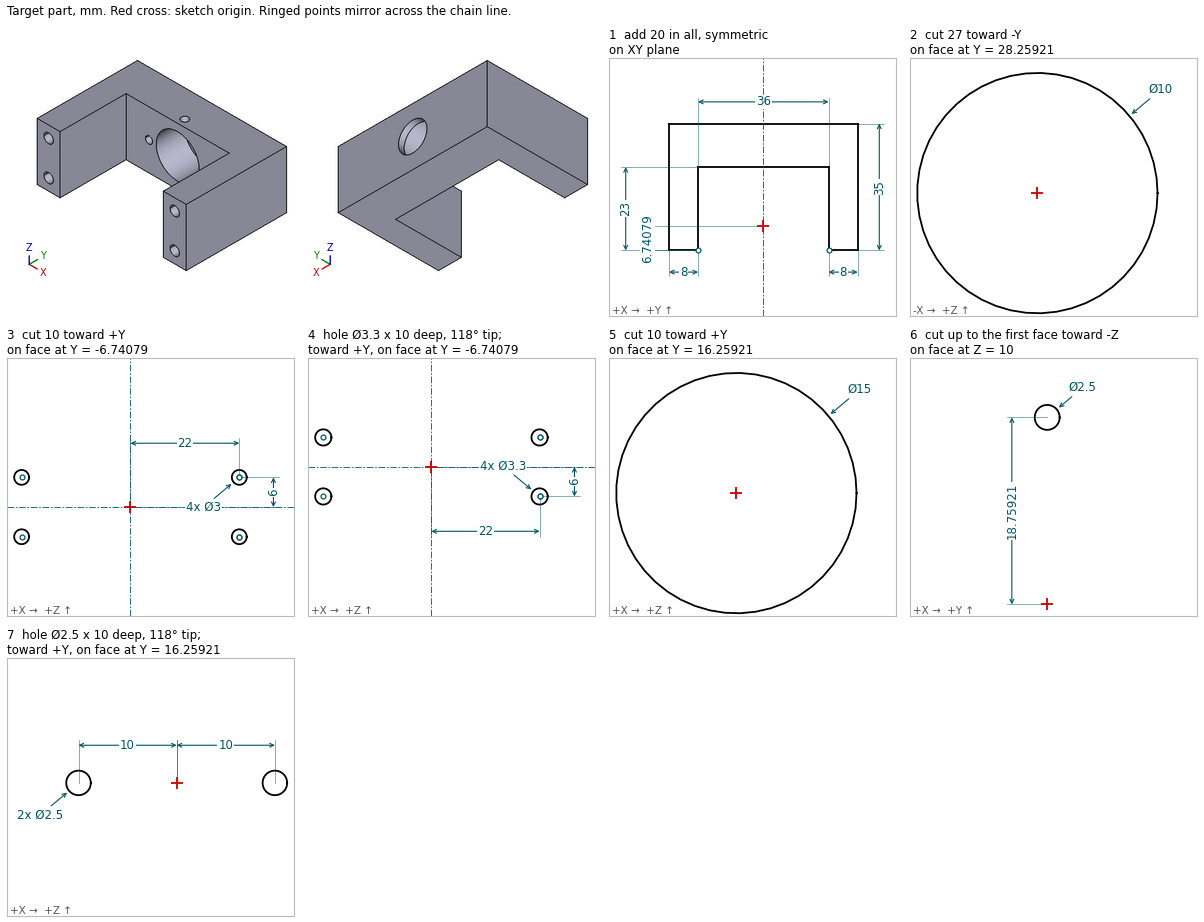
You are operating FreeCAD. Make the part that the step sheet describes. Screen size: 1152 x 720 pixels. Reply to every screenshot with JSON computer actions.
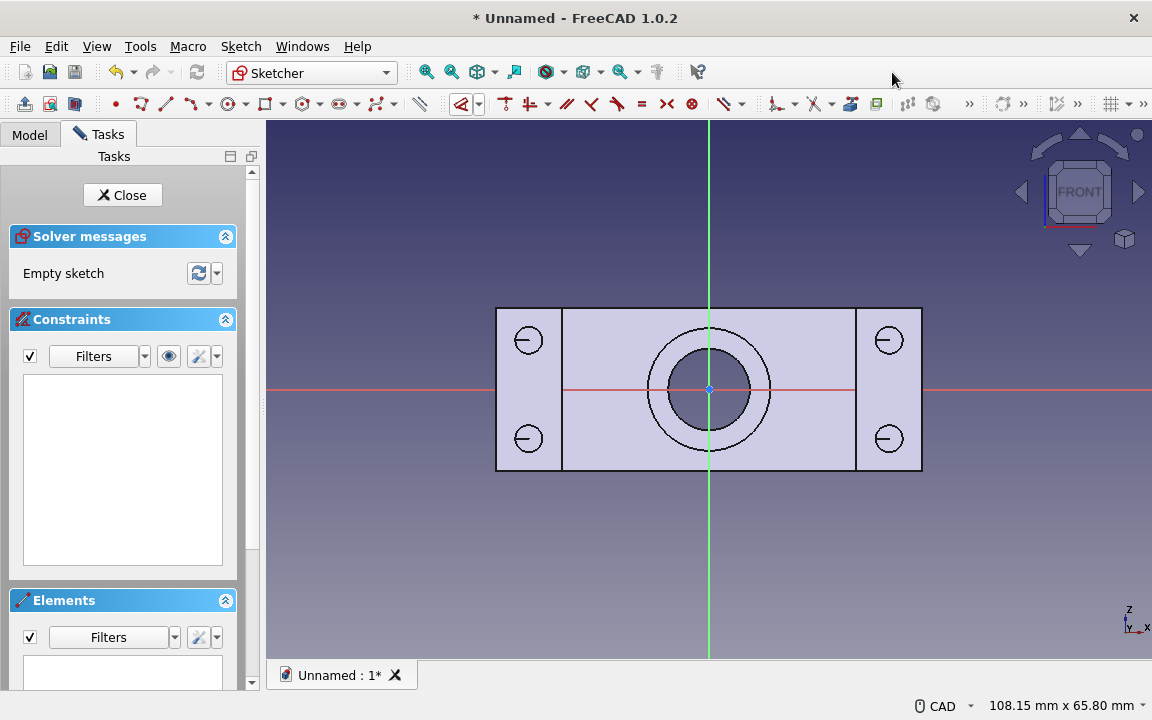
{"action": "key", "text": "q s"}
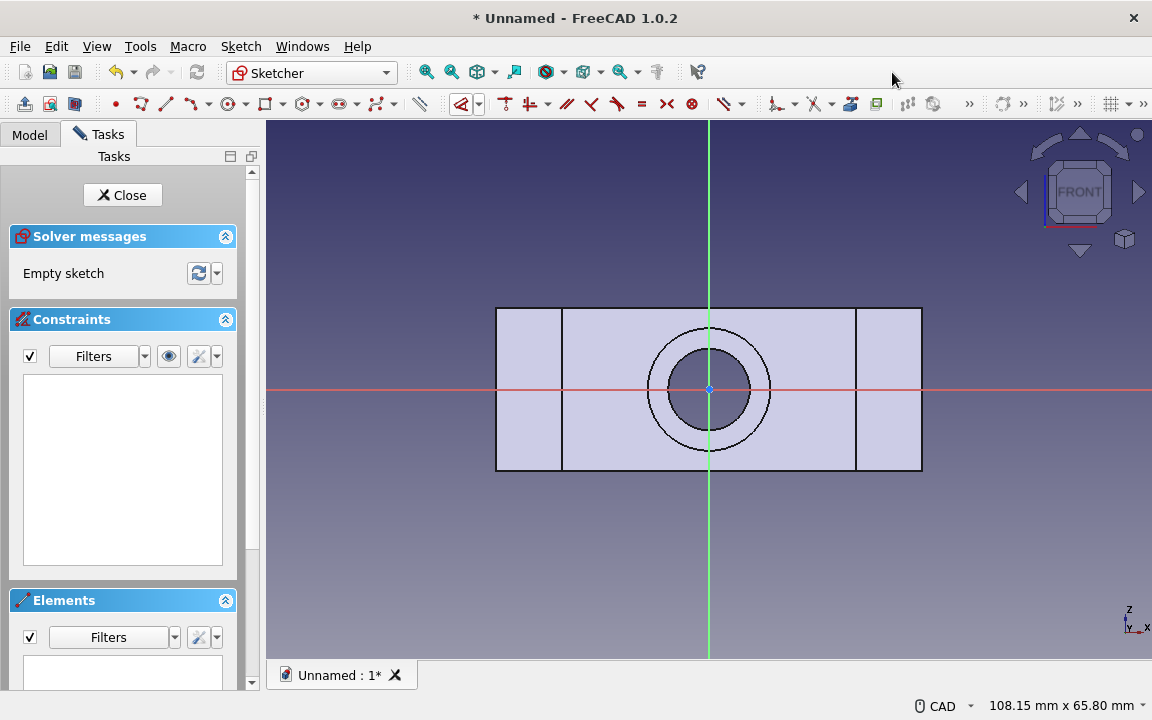
{"action": "scroll", "coordinate": [749, 390], "scroll_direction": "up", "scroll_amount": 5}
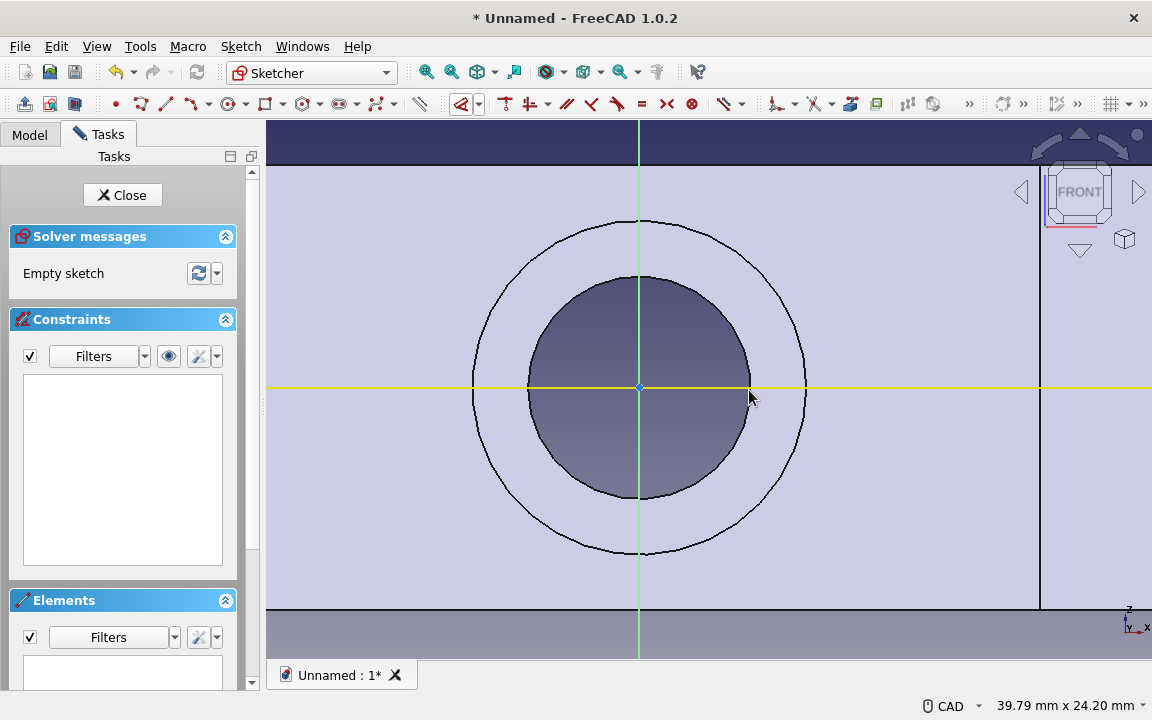
{"action": "key", "text": "g c"}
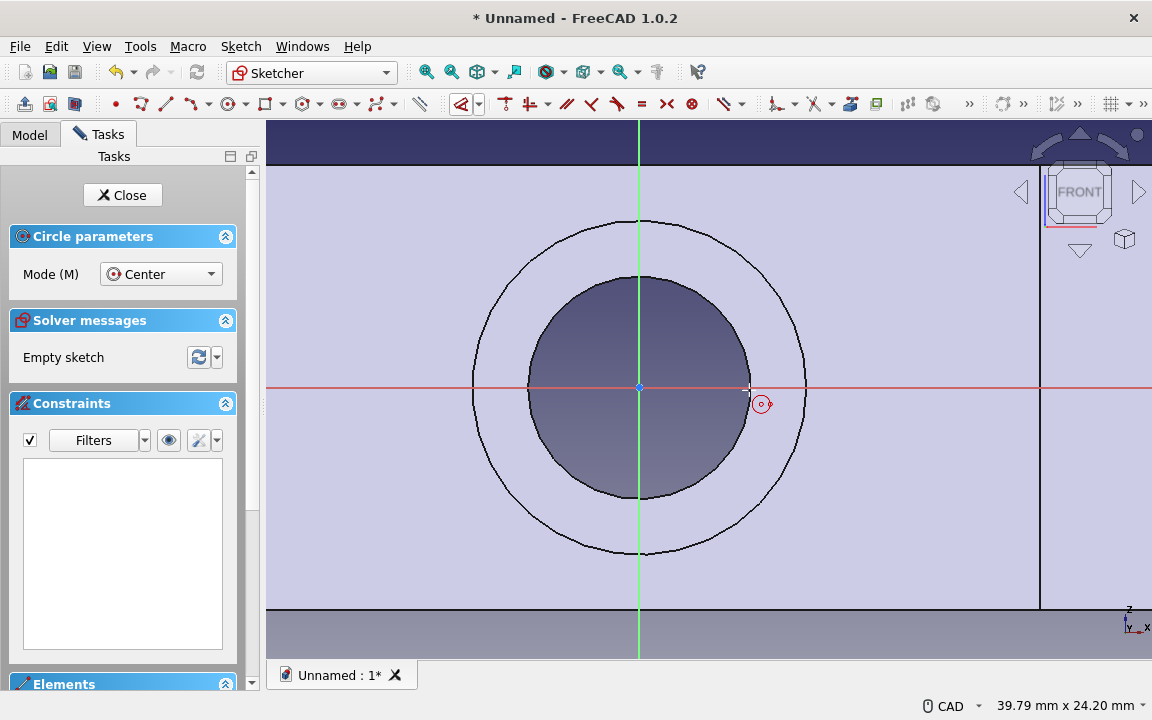
{"action": "left_click", "coordinate": [417, 388]}
{"action": "left_click", "coordinate": [436, 368]}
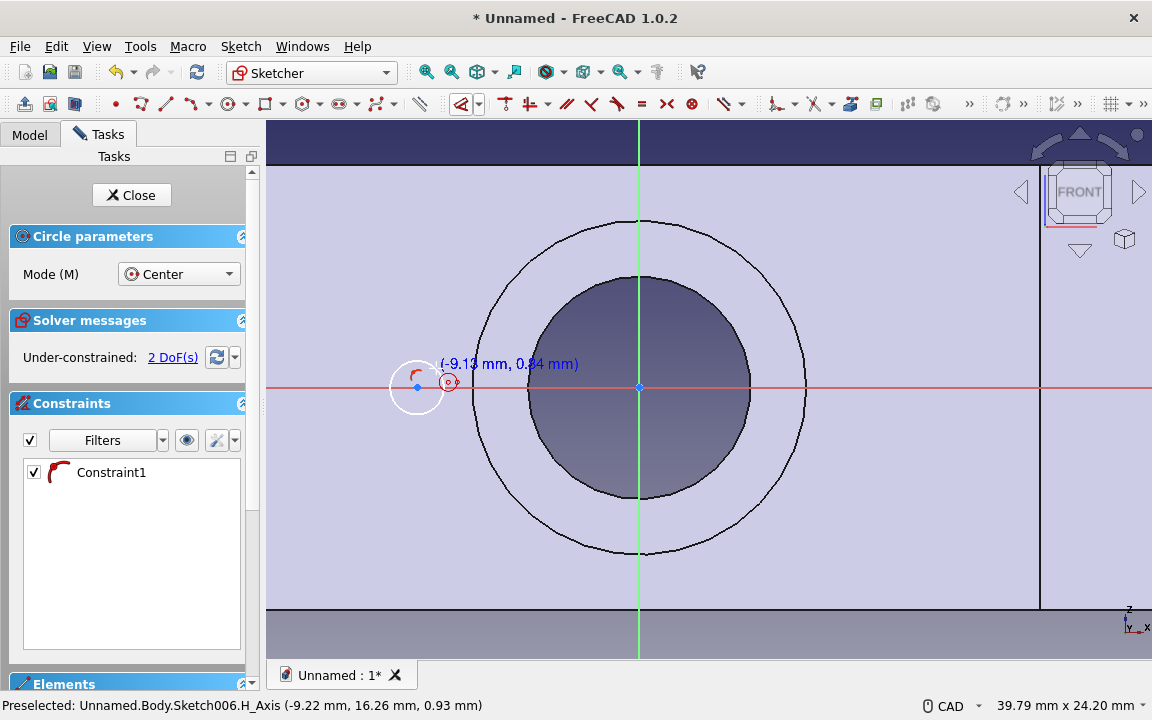
{"action": "left_click", "coordinate": [862, 388]}
{"action": "left_click", "coordinate": [882, 368]}
{"action": "key", "text": "Escape"}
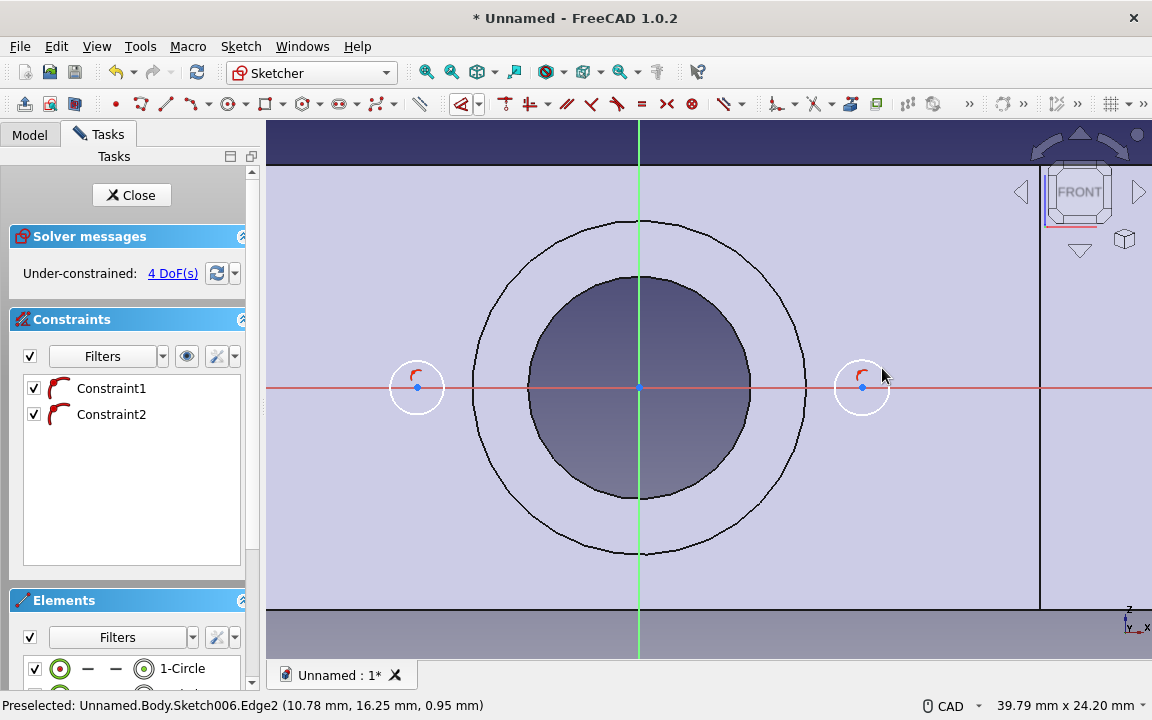
{"action": "left_click", "coordinate": [436, 369]}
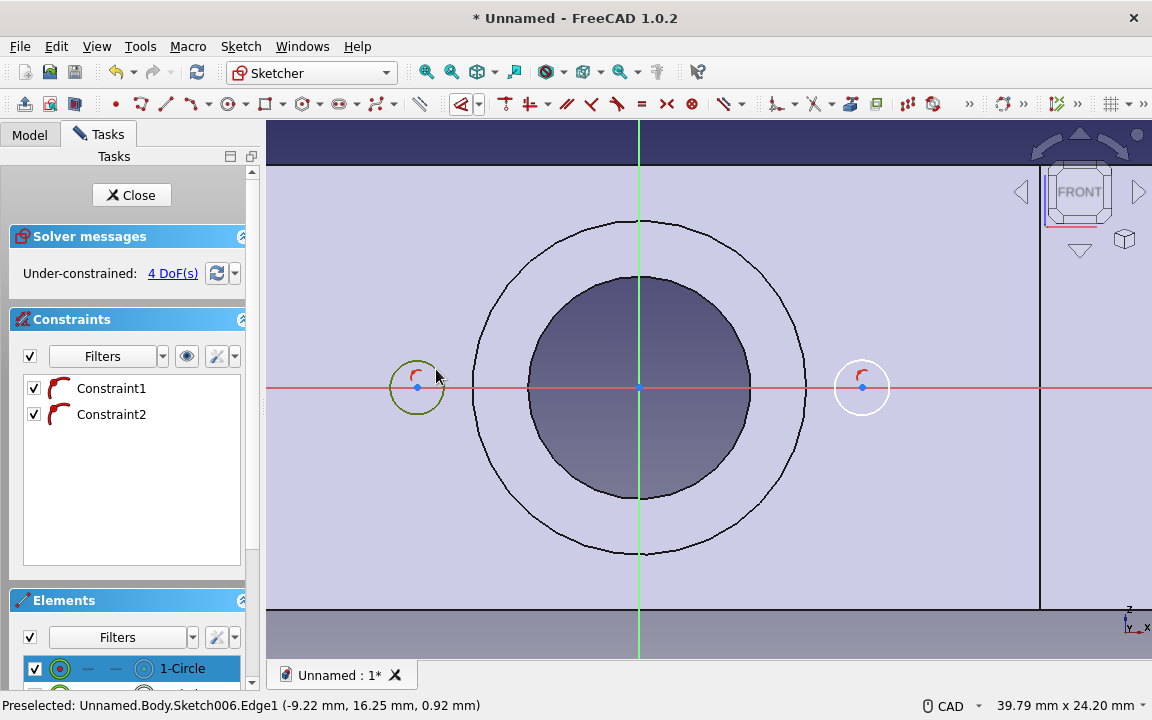
{"action": "left_click", "coordinate": [881, 368]}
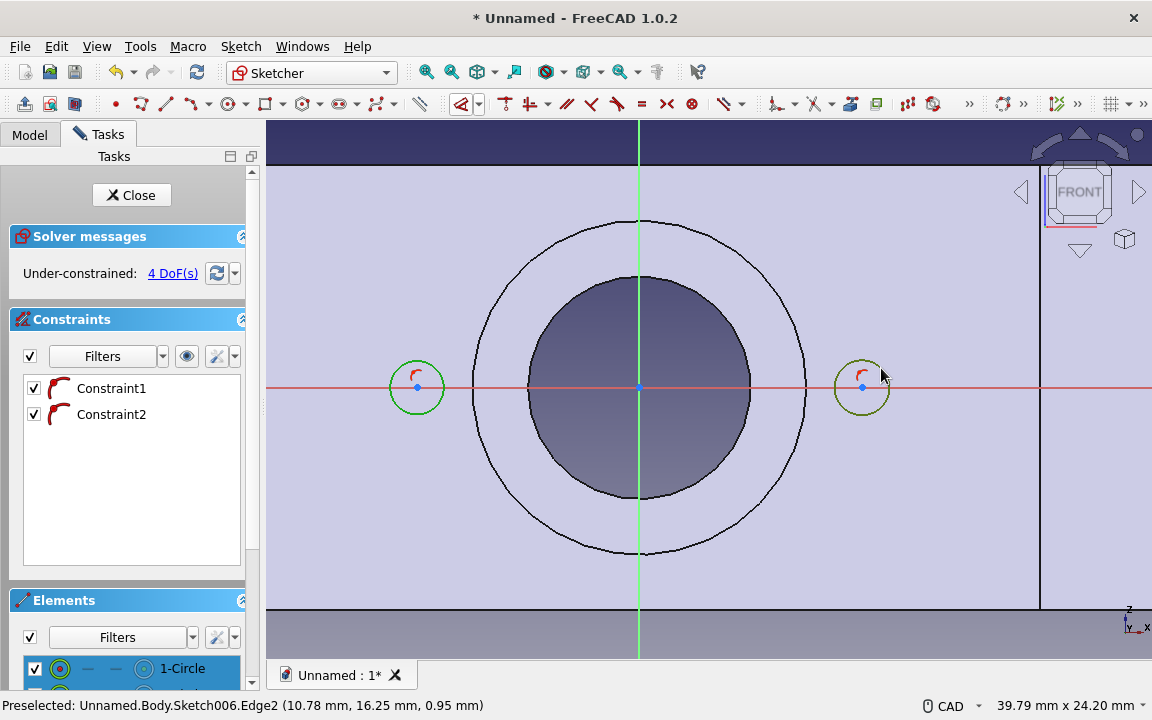
{"action": "key", "text": "e"}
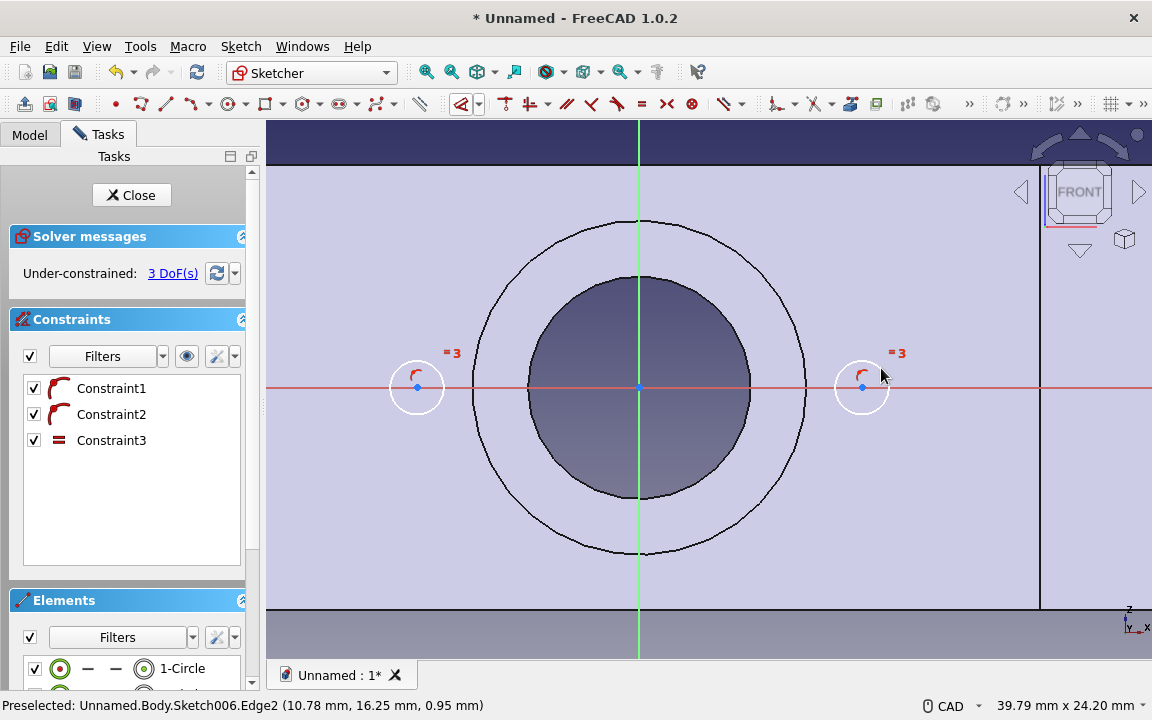
{"action": "left_click", "coordinate": [436, 369]}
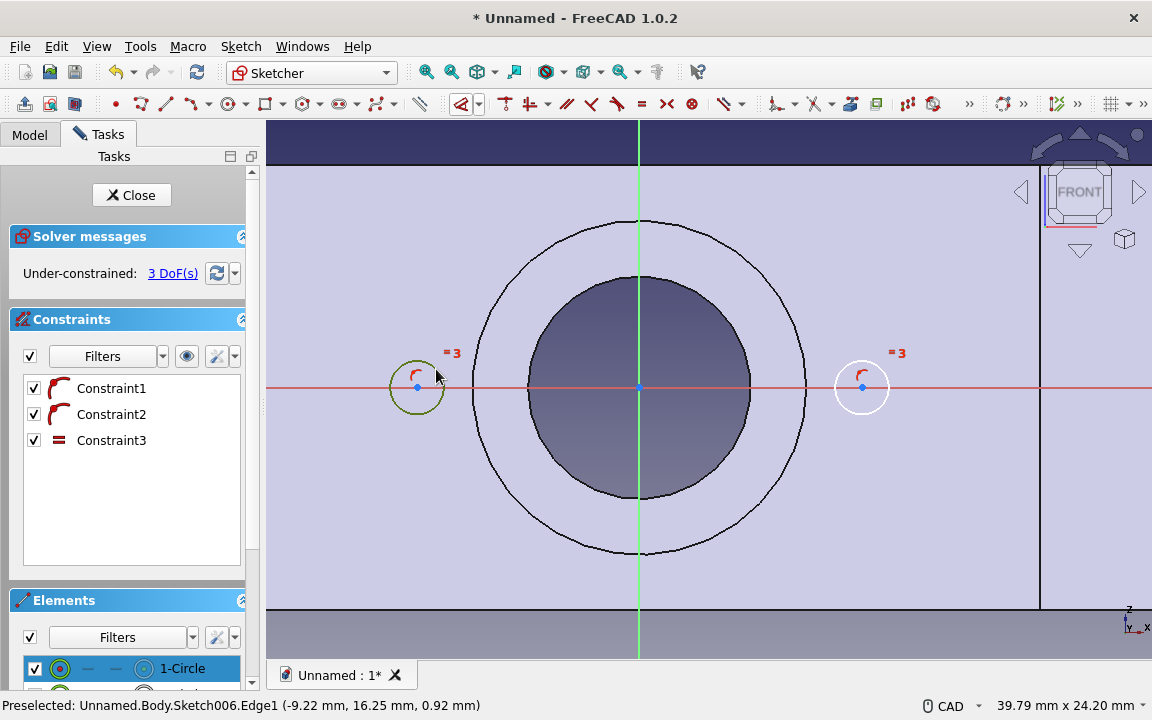
{"action": "key", "text": "k o"}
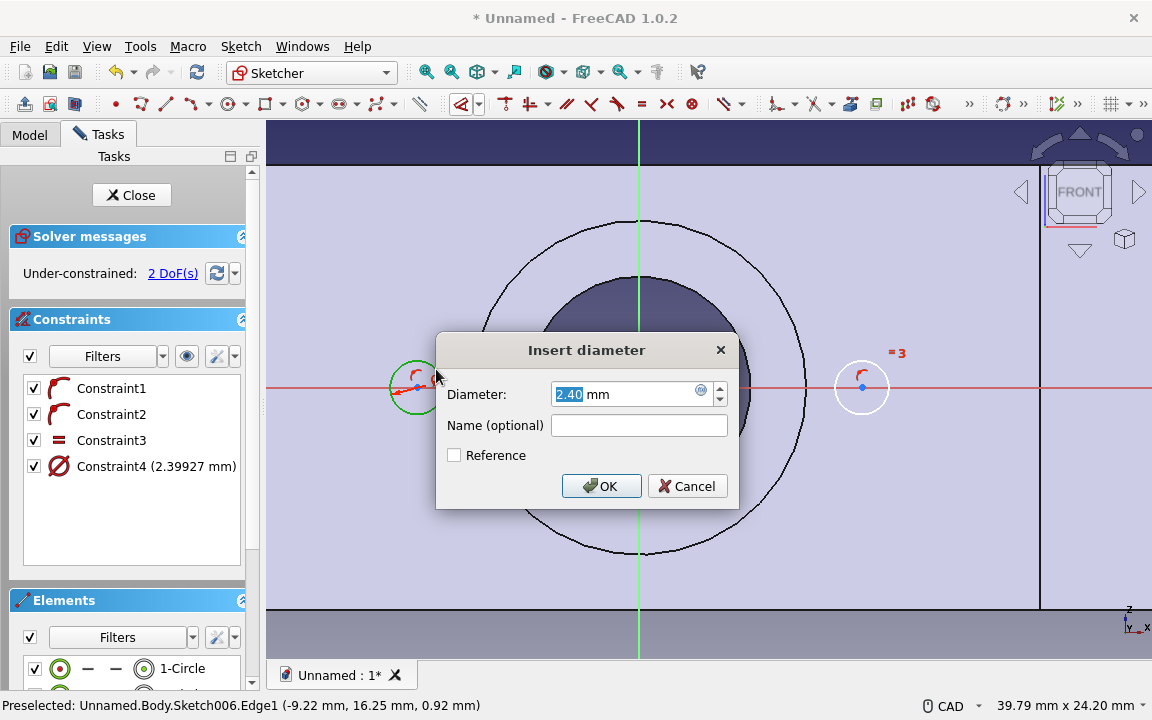
{"action": "type", "text": "2.5"}
{"action": "key", "text": "Return"}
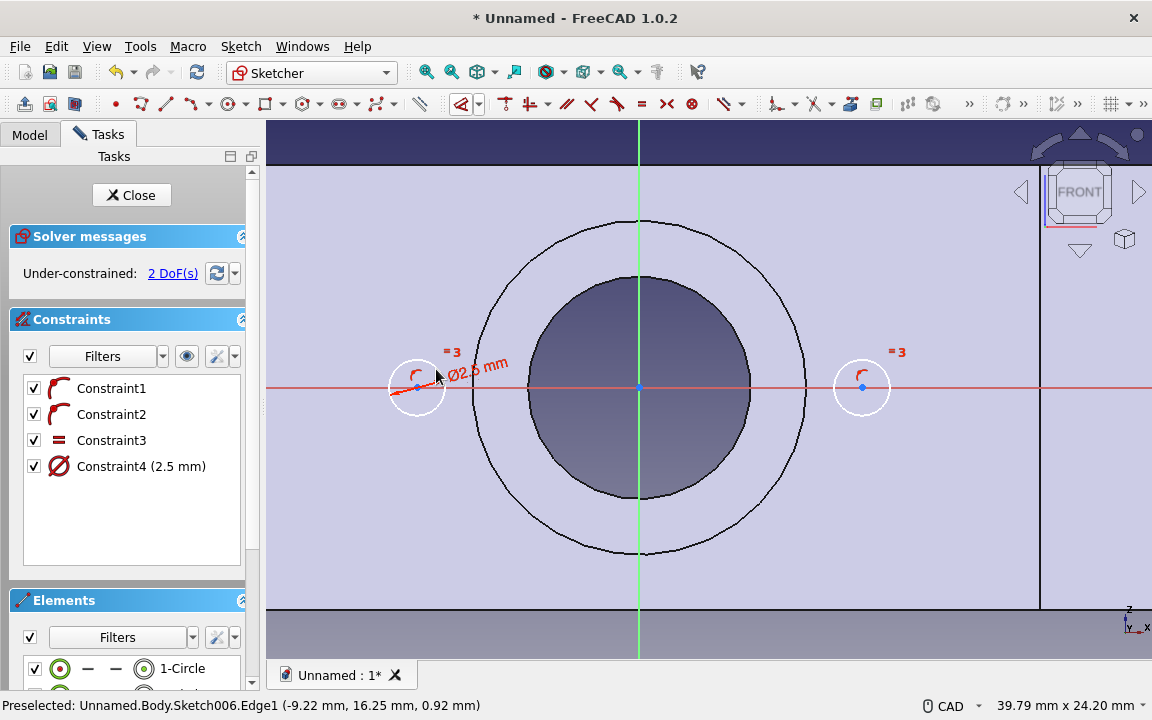
{"action": "left_click", "coordinate": [417, 388]}